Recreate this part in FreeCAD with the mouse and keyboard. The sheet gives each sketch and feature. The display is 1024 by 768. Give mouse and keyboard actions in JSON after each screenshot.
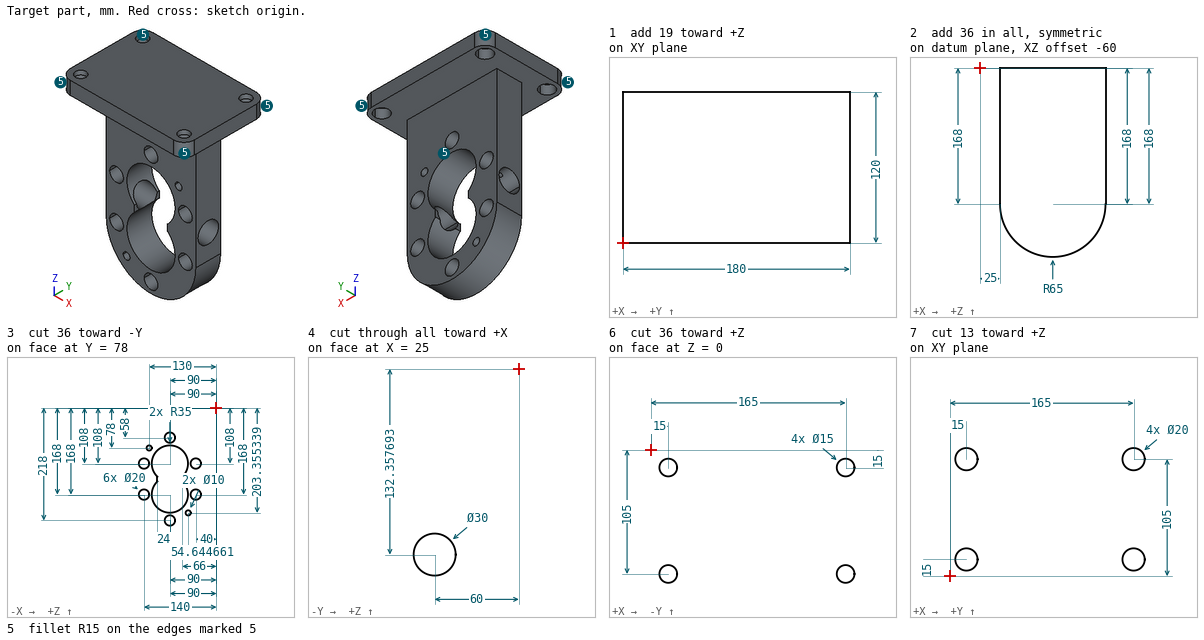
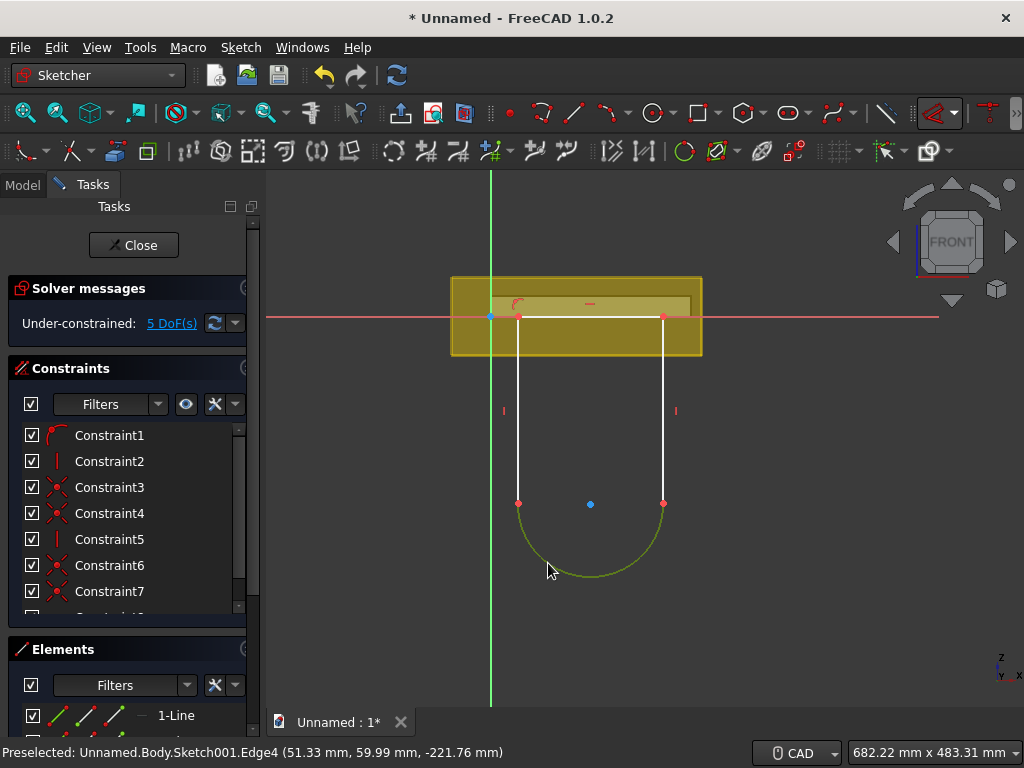
{"action": "key", "text": "k r"}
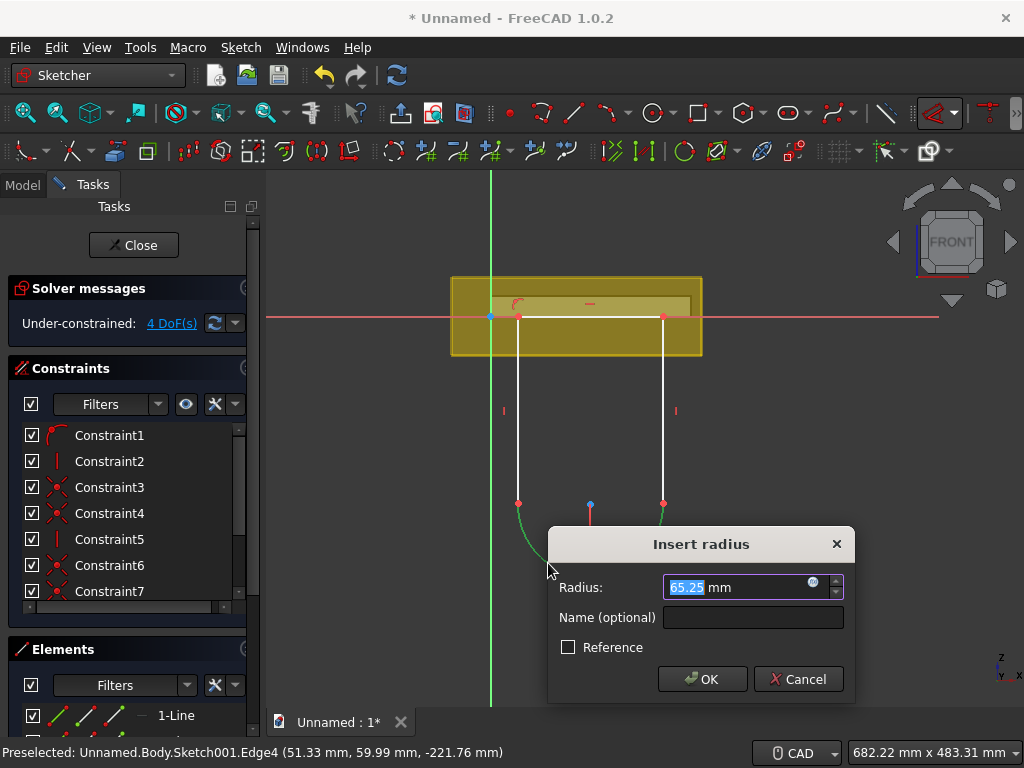
{"action": "type", "text": "65"}
{"action": "key", "text": "Return"}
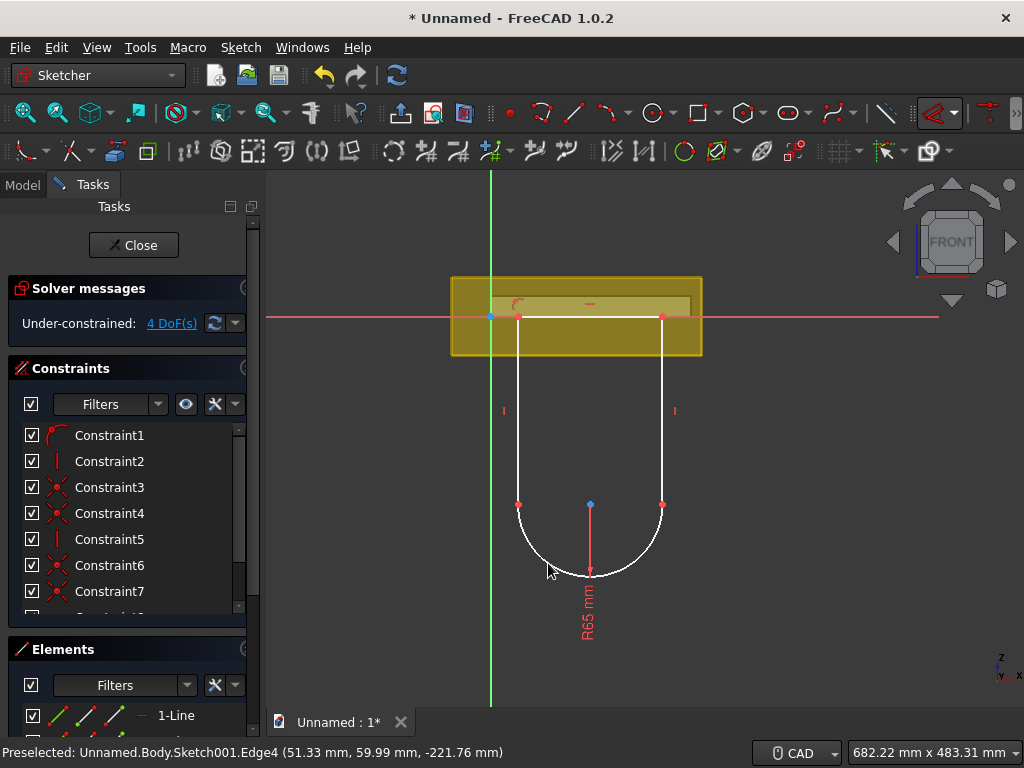
{"action": "left_click", "coordinate": [518, 448]}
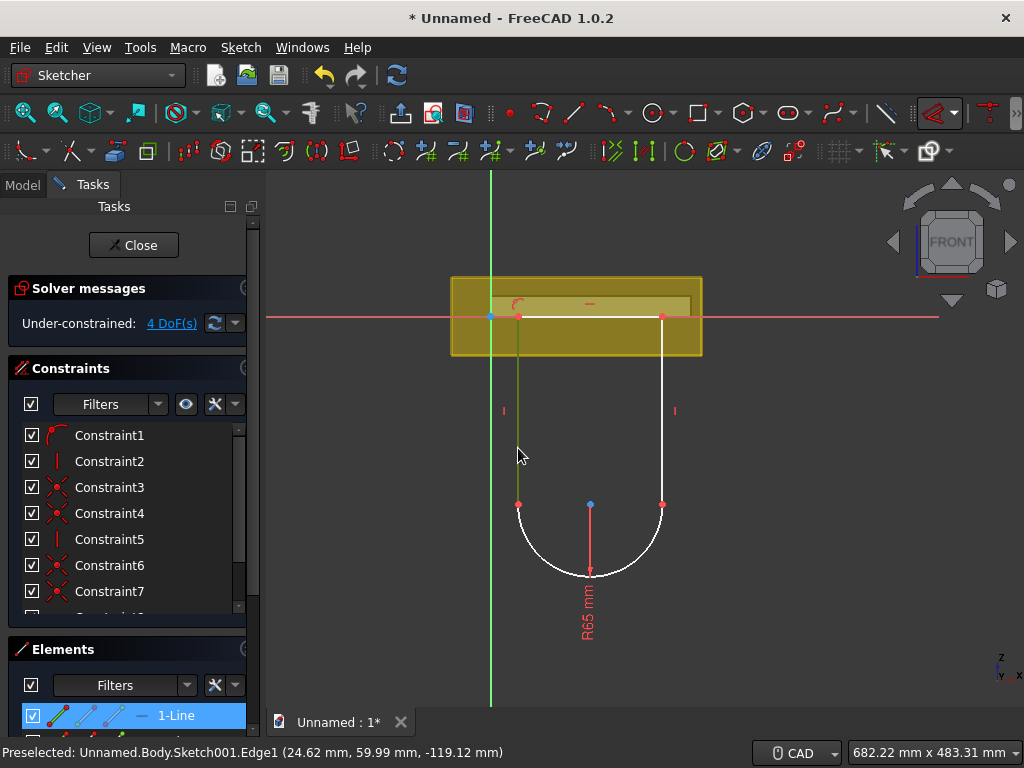
{"action": "left_click", "coordinate": [956, 114]}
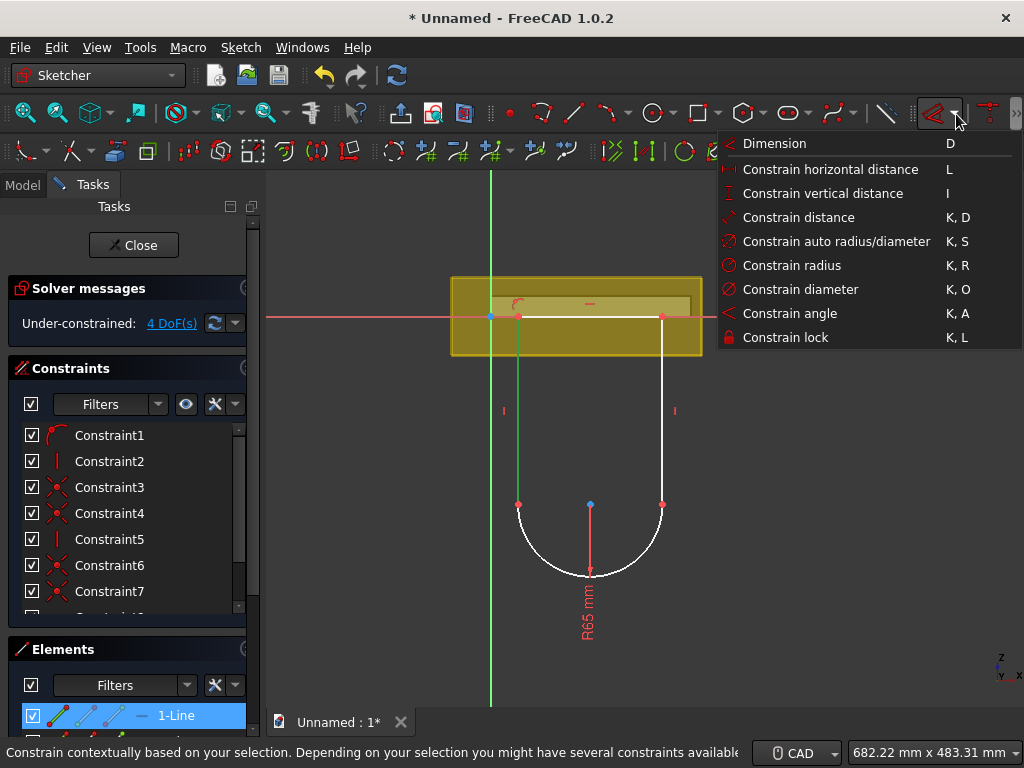
{"action": "left_click", "coordinate": [870, 193]}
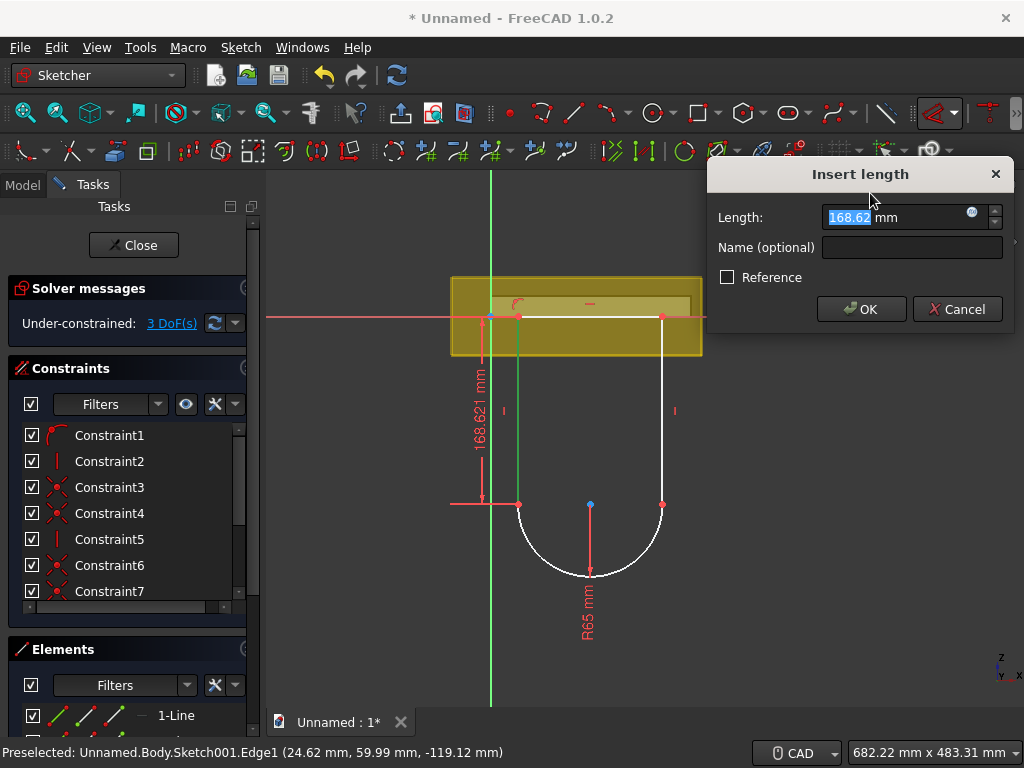
{"action": "type", "text": "168"}
{"action": "key", "text": "Return"}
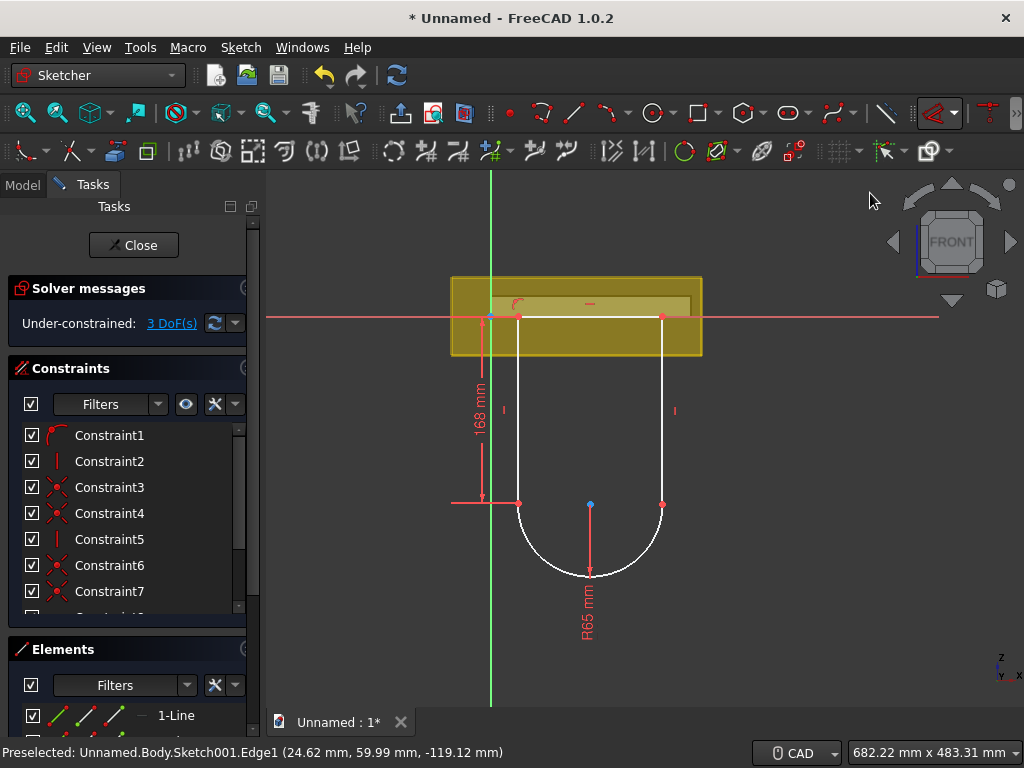
{"action": "left_click", "coordinate": [662, 373]}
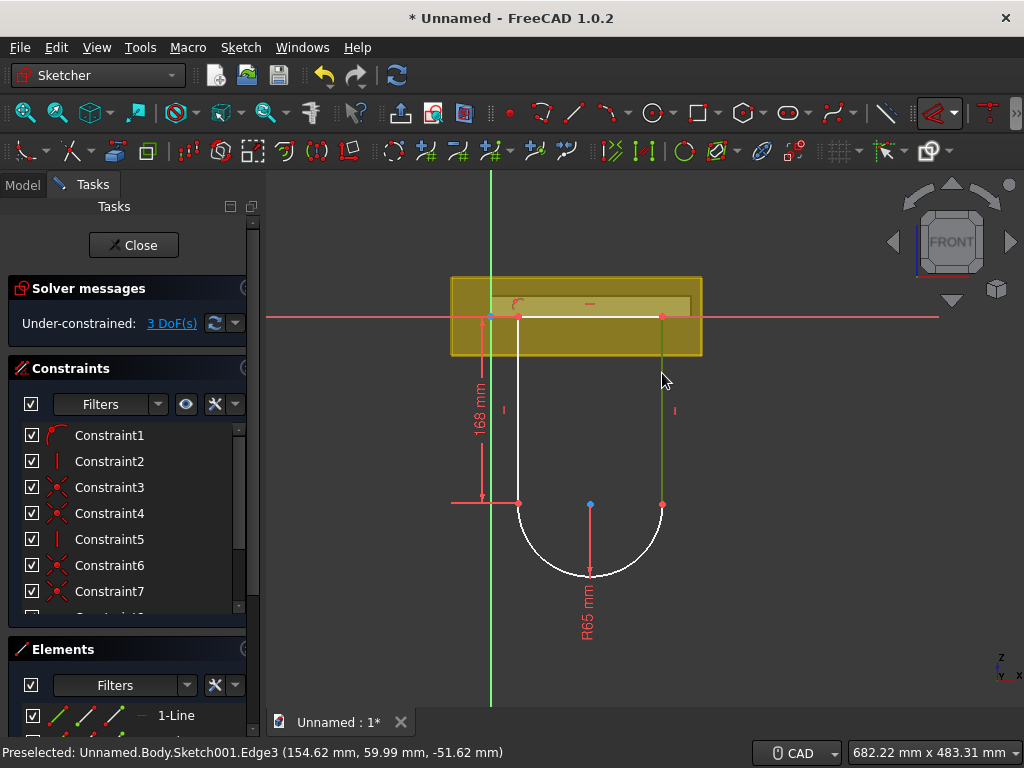
{"action": "left_click", "coordinate": [956, 114]}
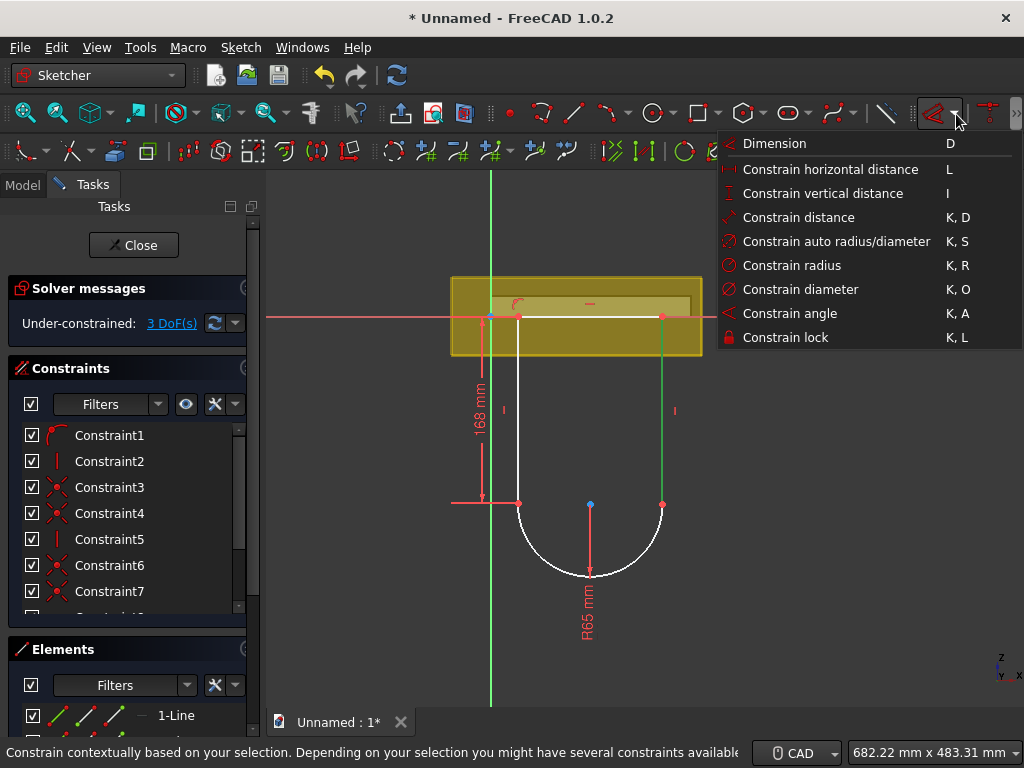
{"action": "left_click", "coordinate": [870, 193]}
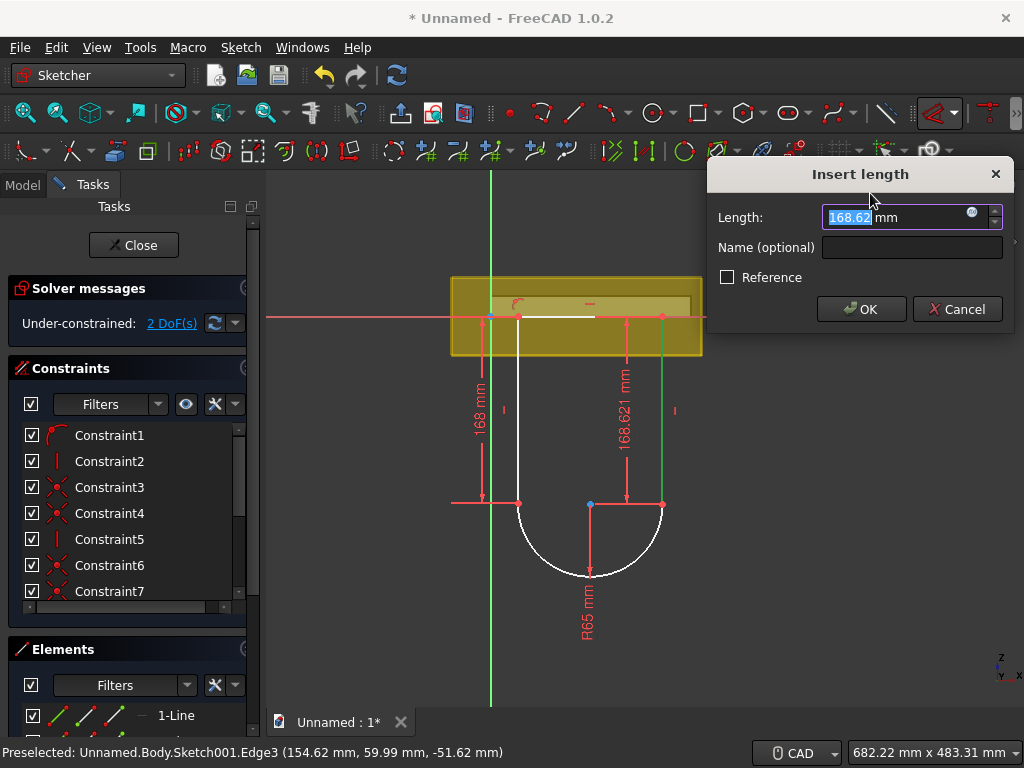
{"action": "type", "text": "168"}
{"action": "key", "text": "Return"}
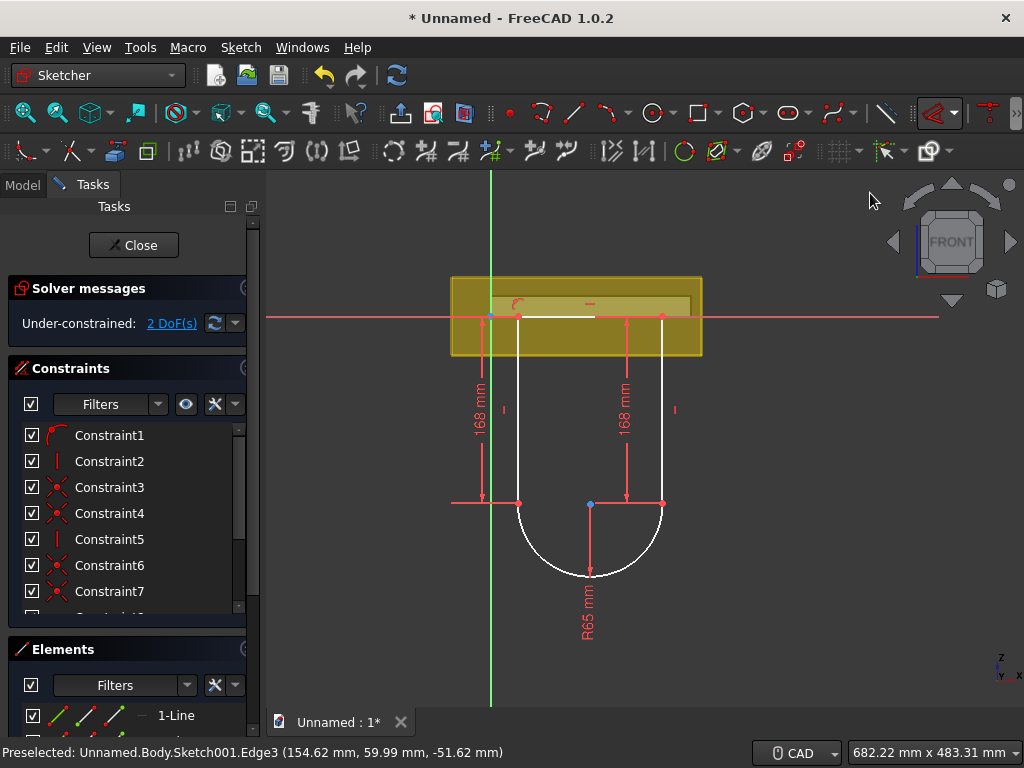
{"action": "scroll", "coordinate": [518, 503], "scroll_direction": "up", "scroll_amount": 2}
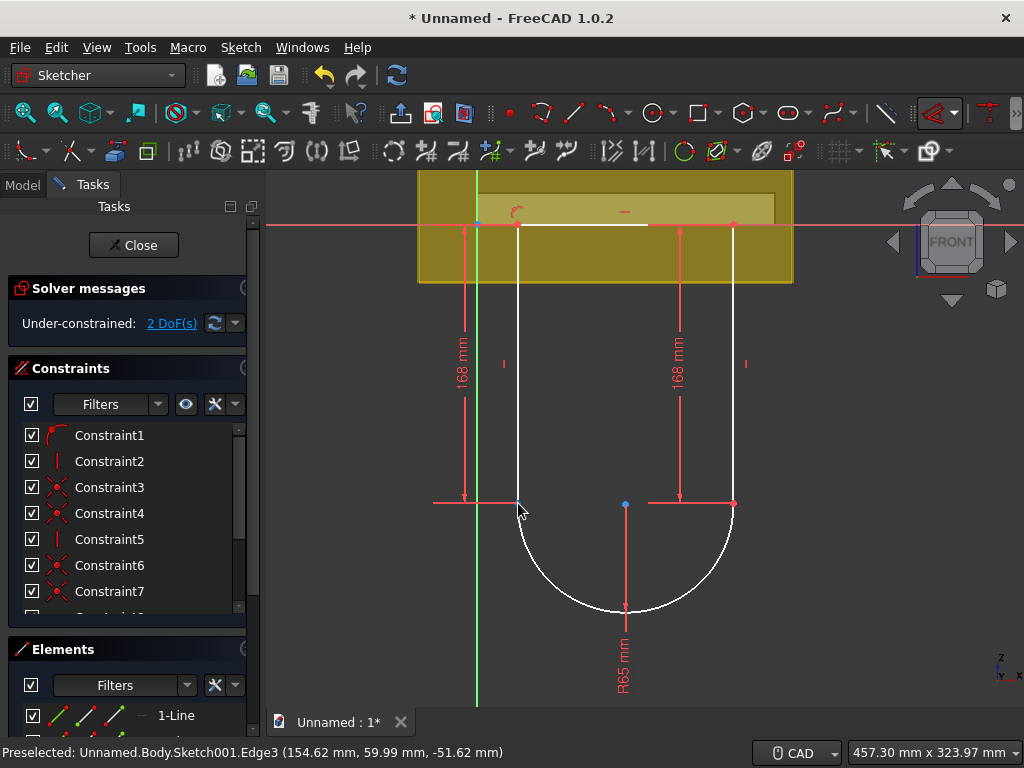
{"action": "left_click", "coordinate": [518, 503]}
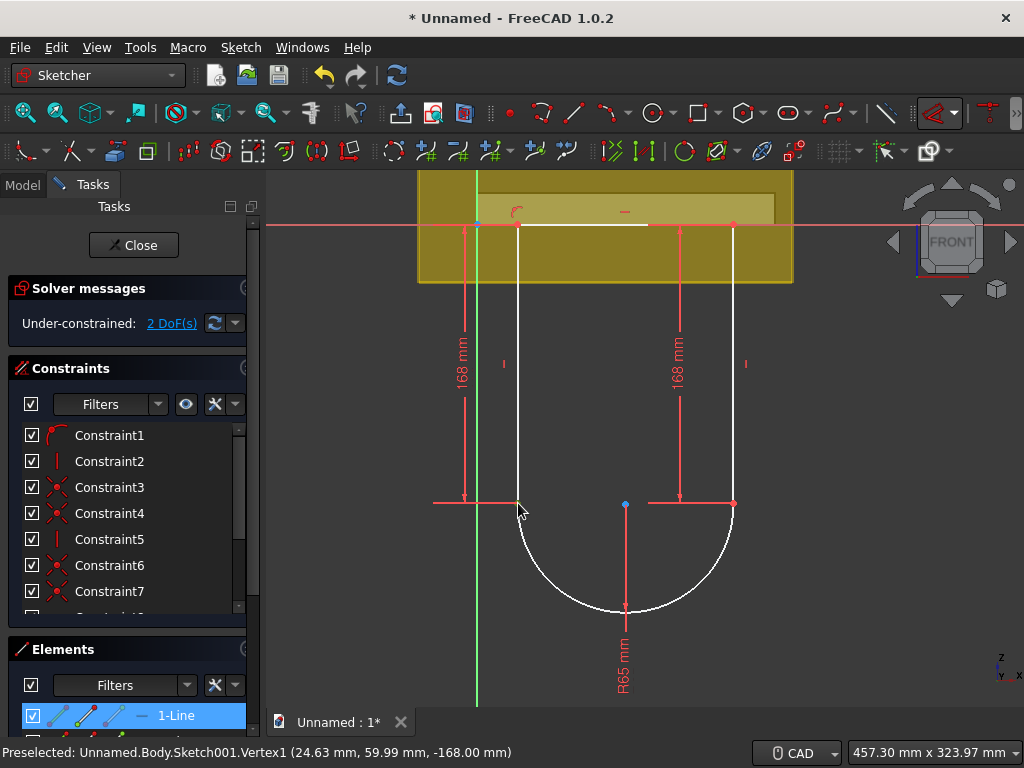
{"action": "key", "text": "l"}